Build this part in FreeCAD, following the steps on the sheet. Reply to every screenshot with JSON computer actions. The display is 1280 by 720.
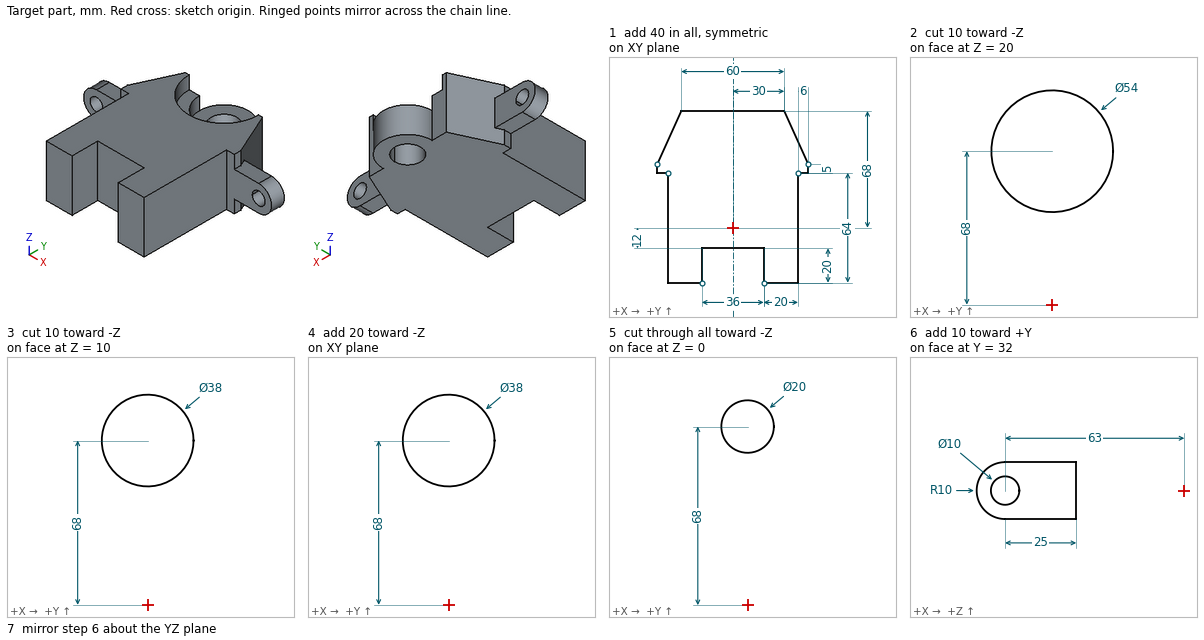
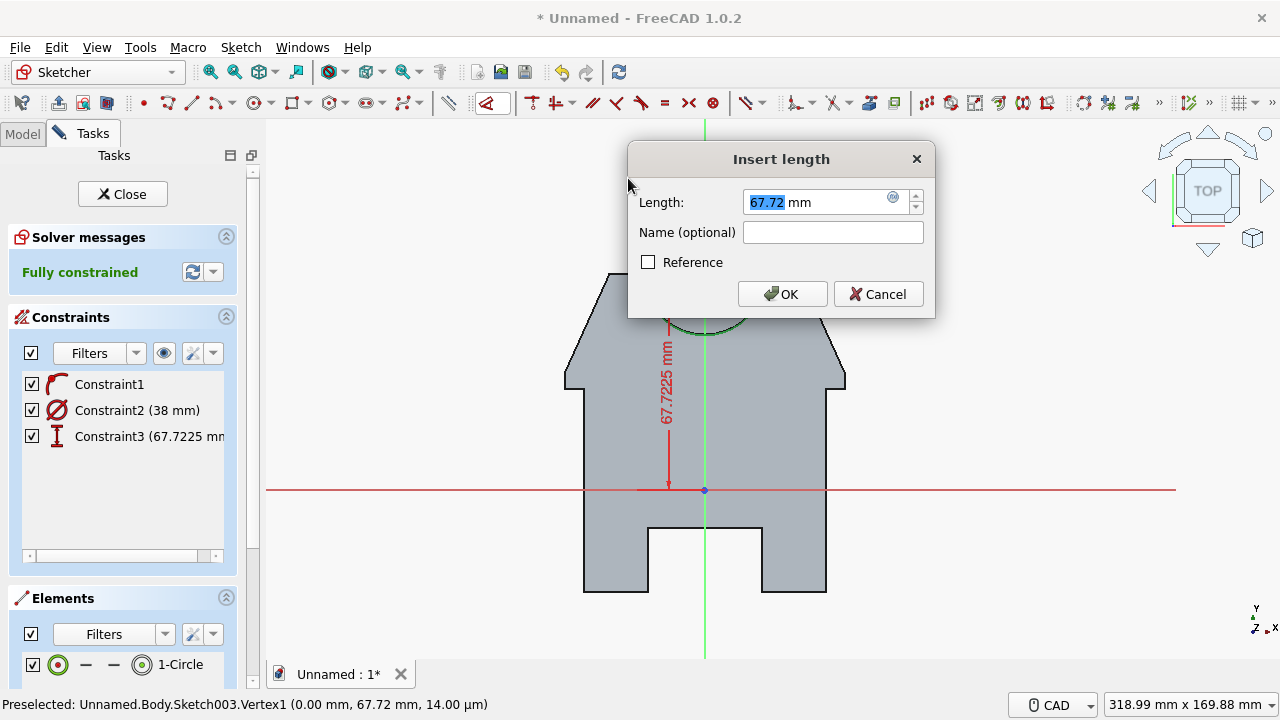
{"action": "type", "text": "68"}
{"action": "key", "text": "Return"}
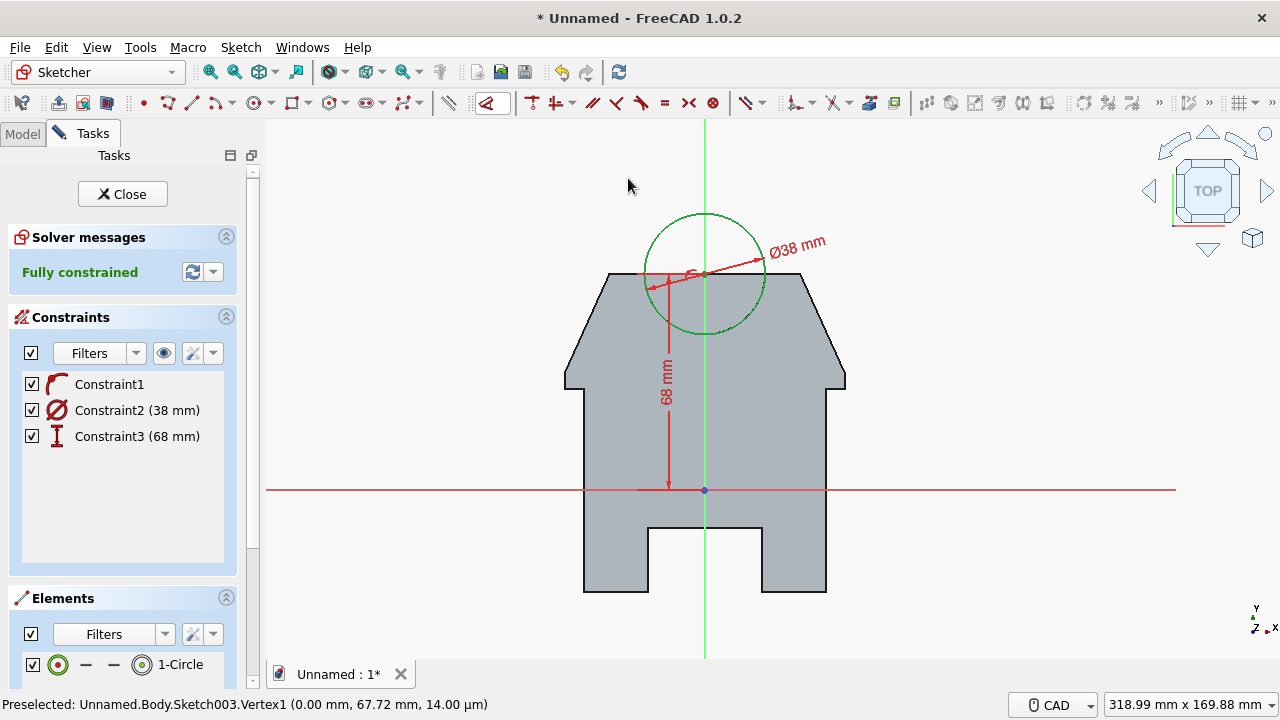
{"action": "left_click", "coordinate": [123, 194]}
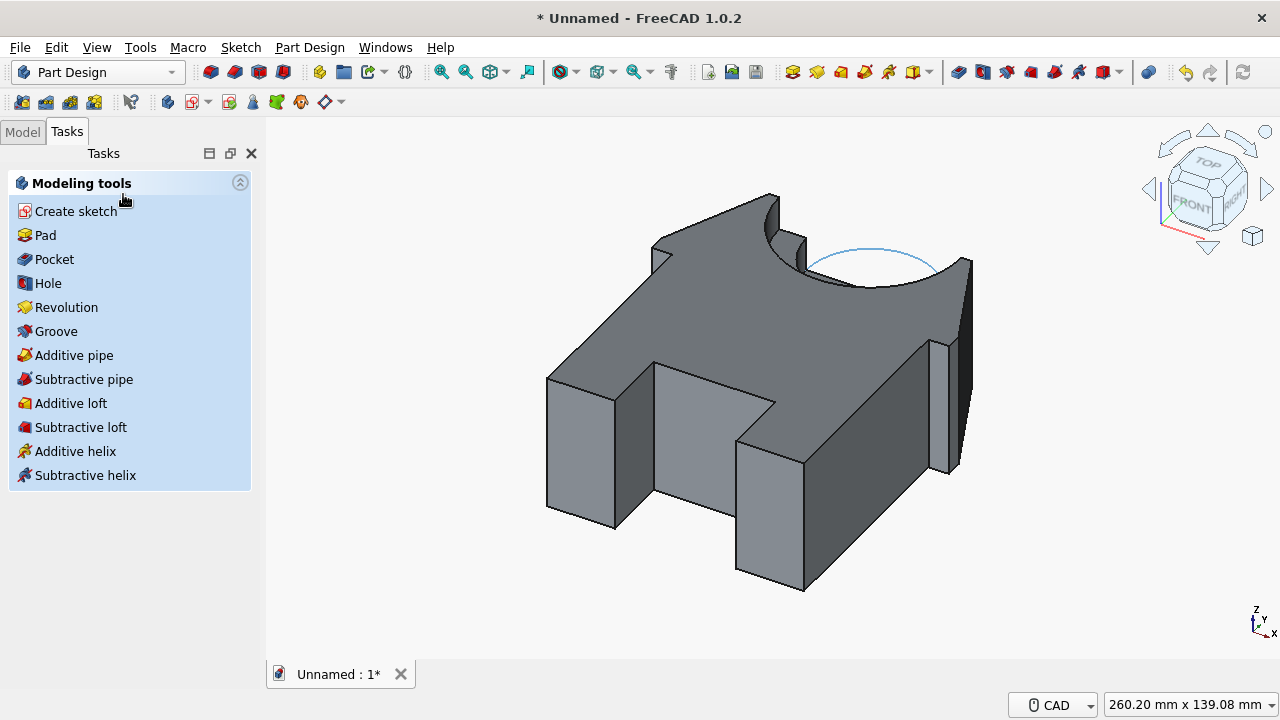
{"action": "left_click", "coordinate": [794, 72]}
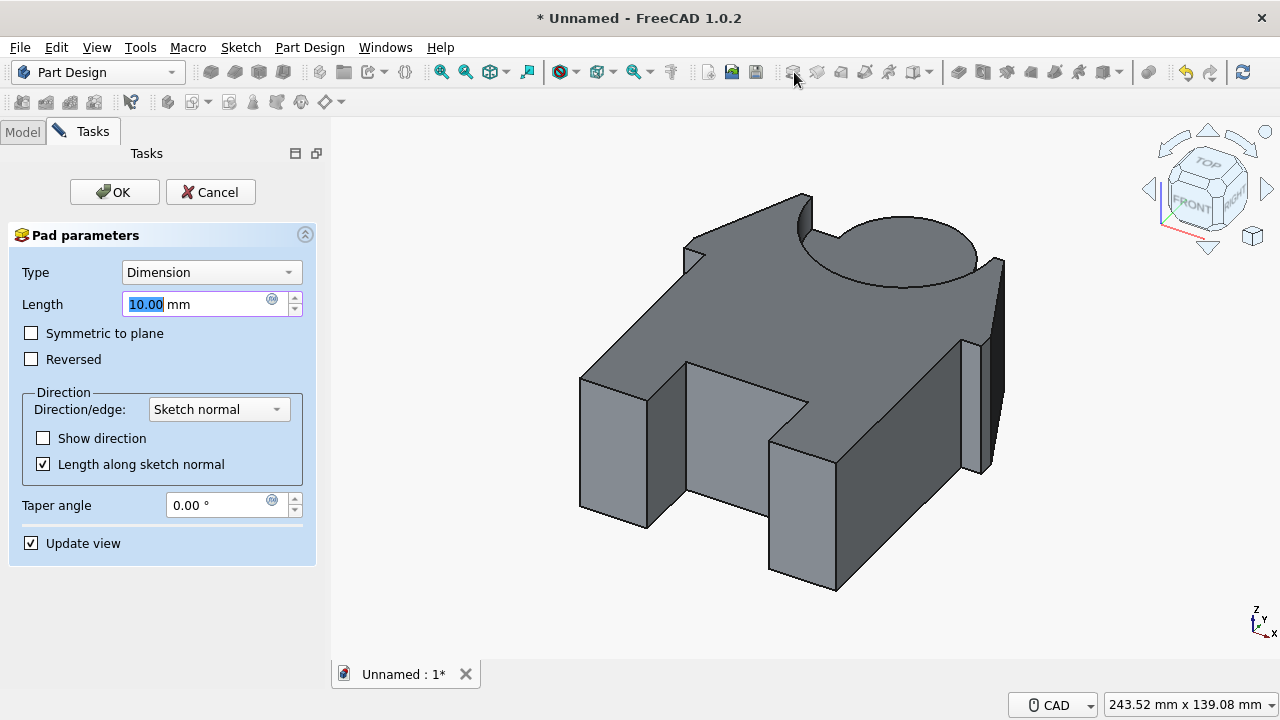
{"action": "type", "text": "20"}
{"action": "key", "text": "Tab"}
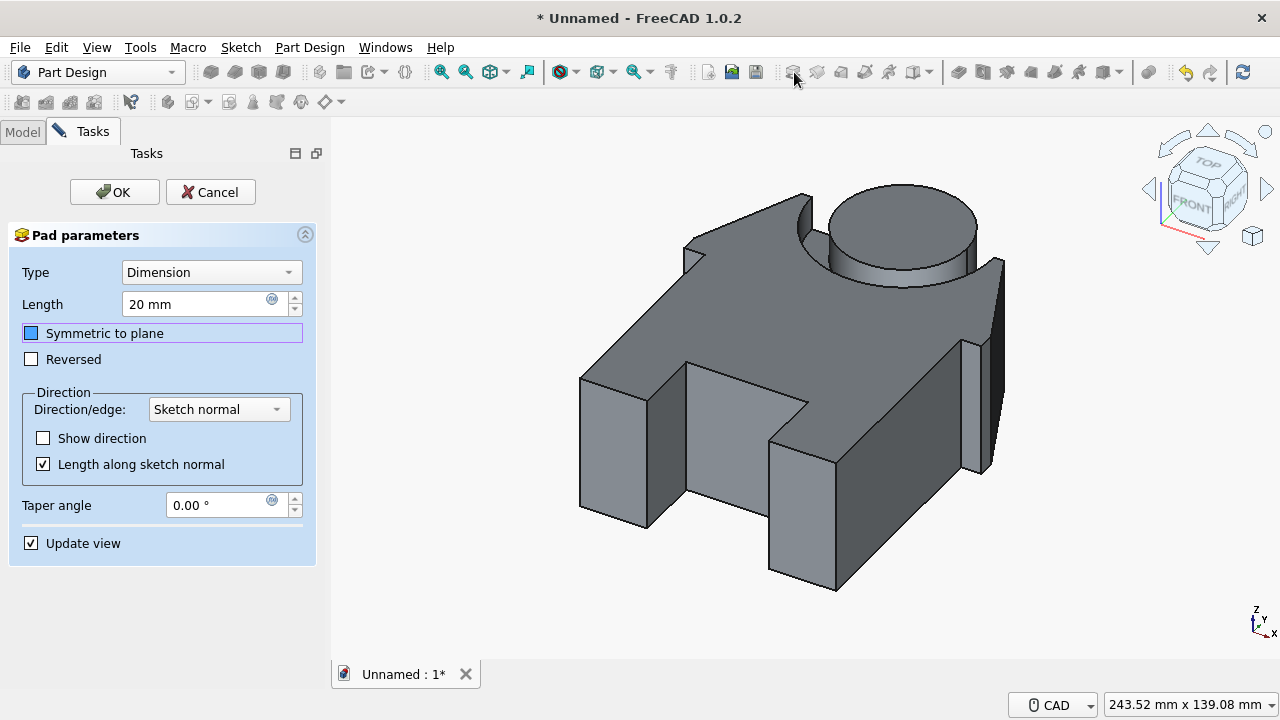
{"action": "left_click", "coordinate": [30, 359]}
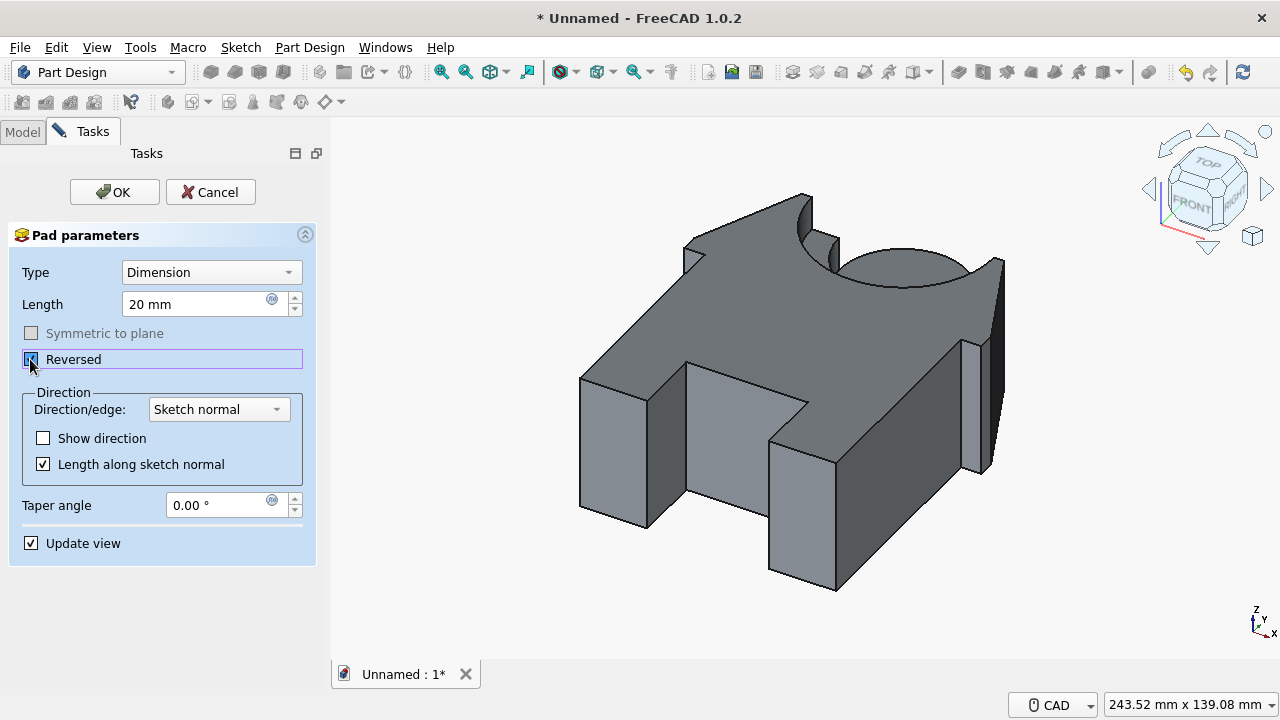
{"action": "left_click", "coordinate": [115, 192]}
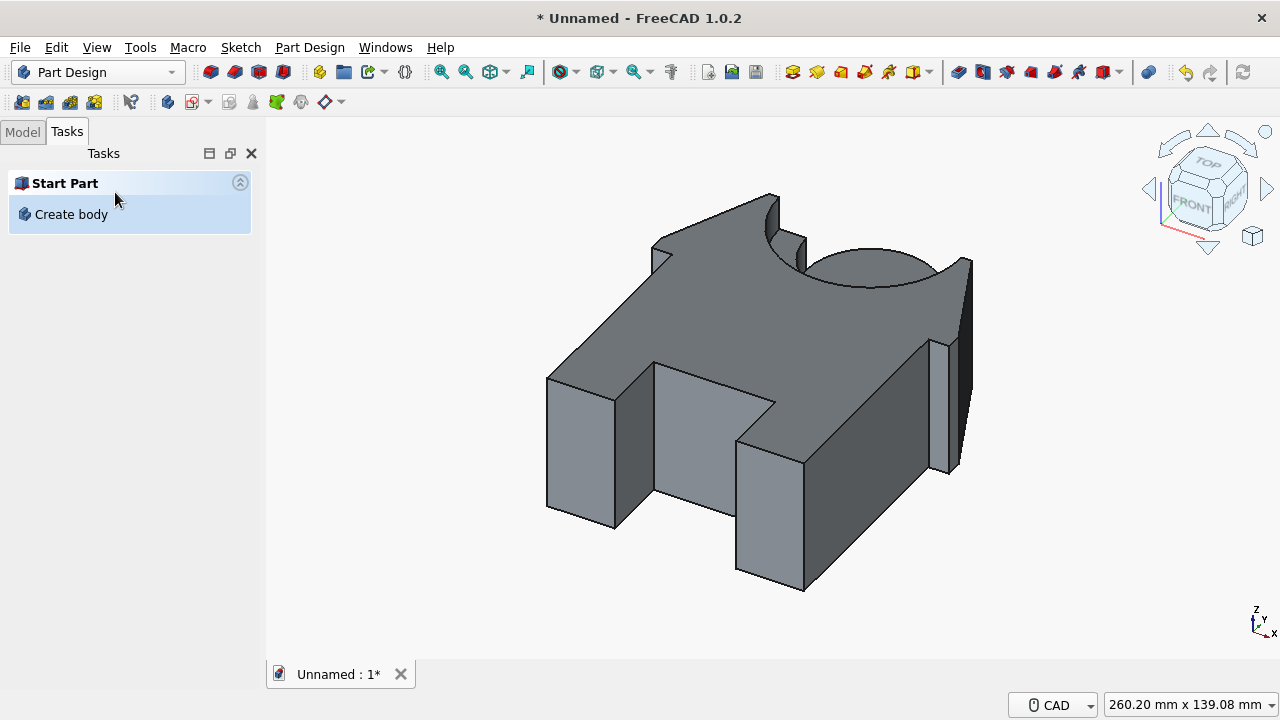
{"action": "key", "text": "0"}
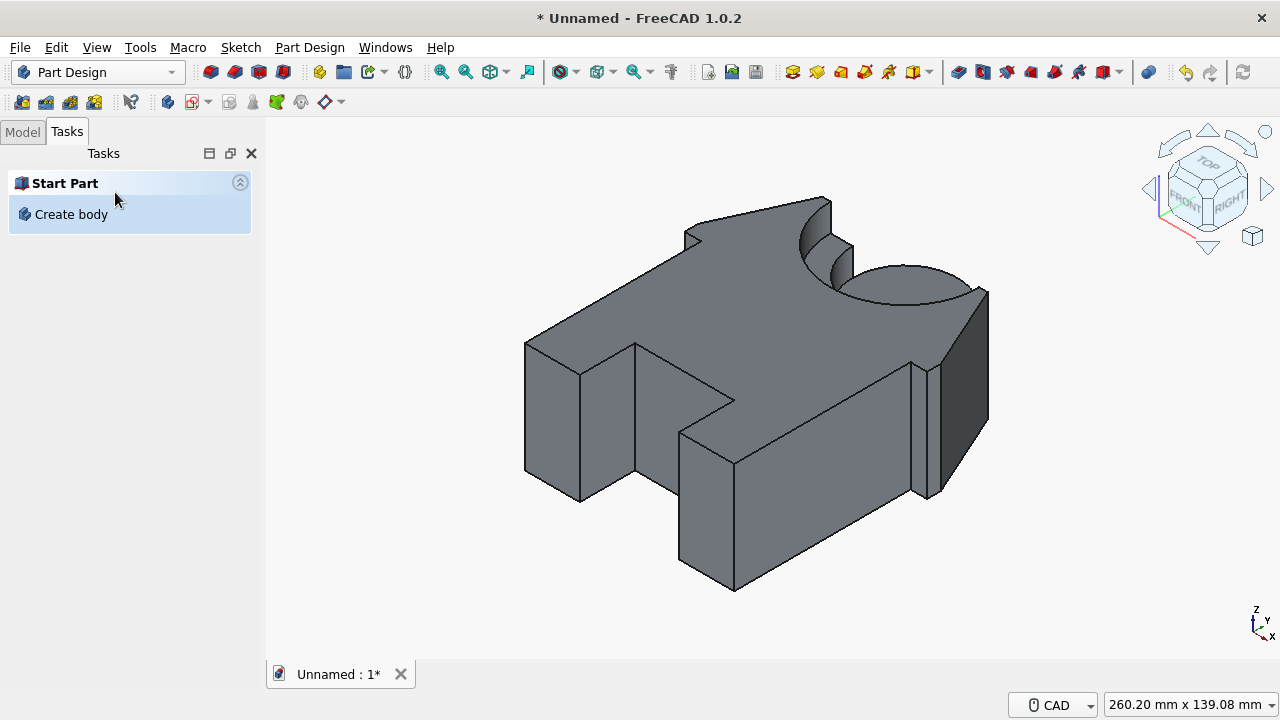
{"action": "key", "text": "2"}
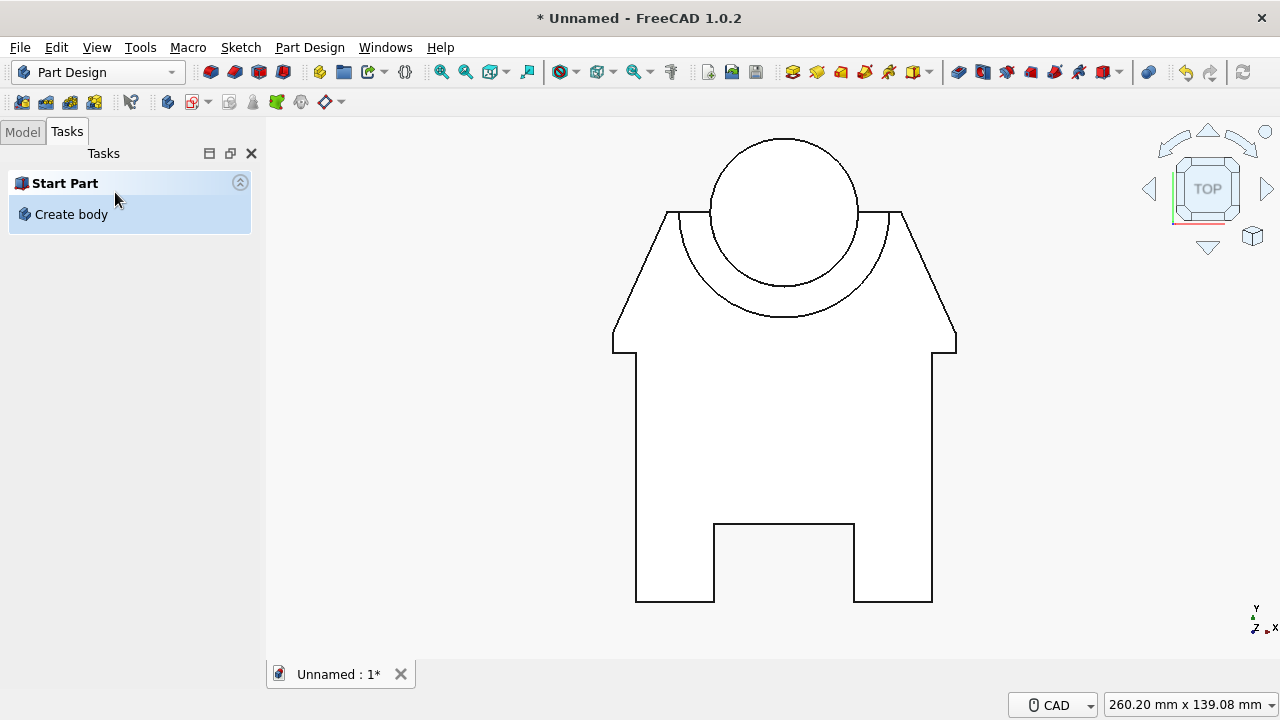
{"action": "left_click", "coordinate": [784, 211]}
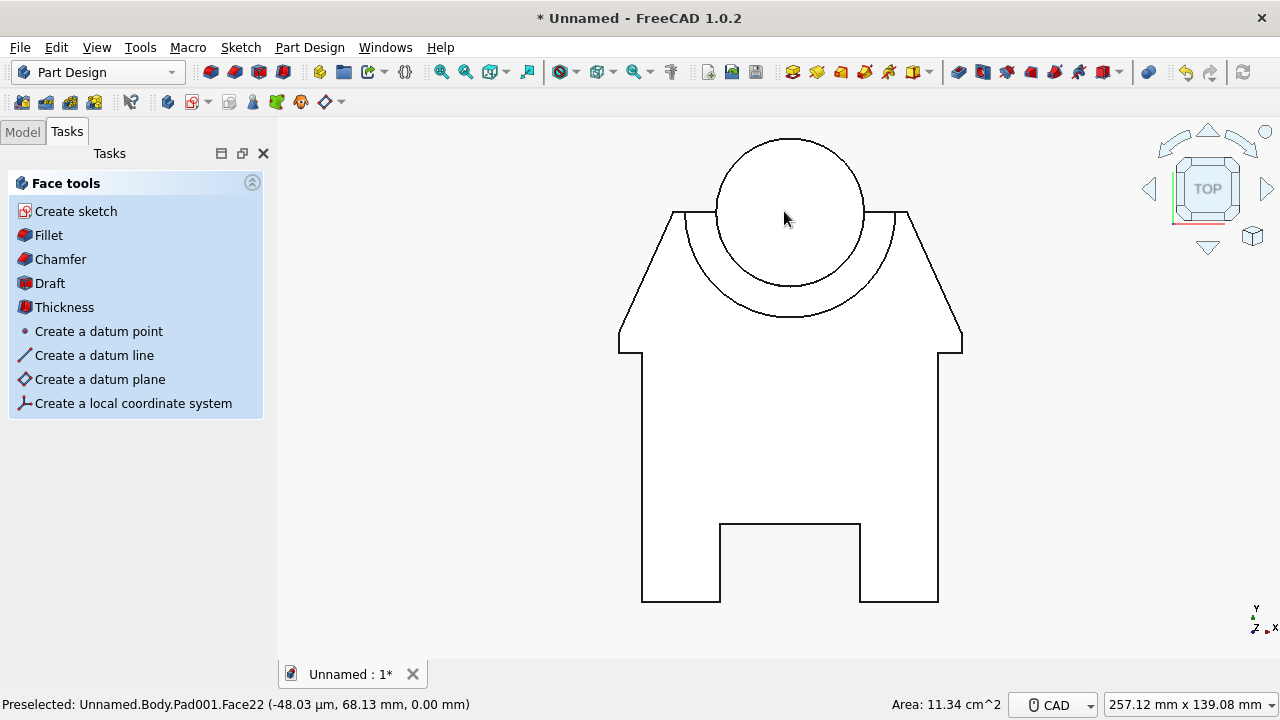
{"action": "left_click", "coordinate": [192, 102]}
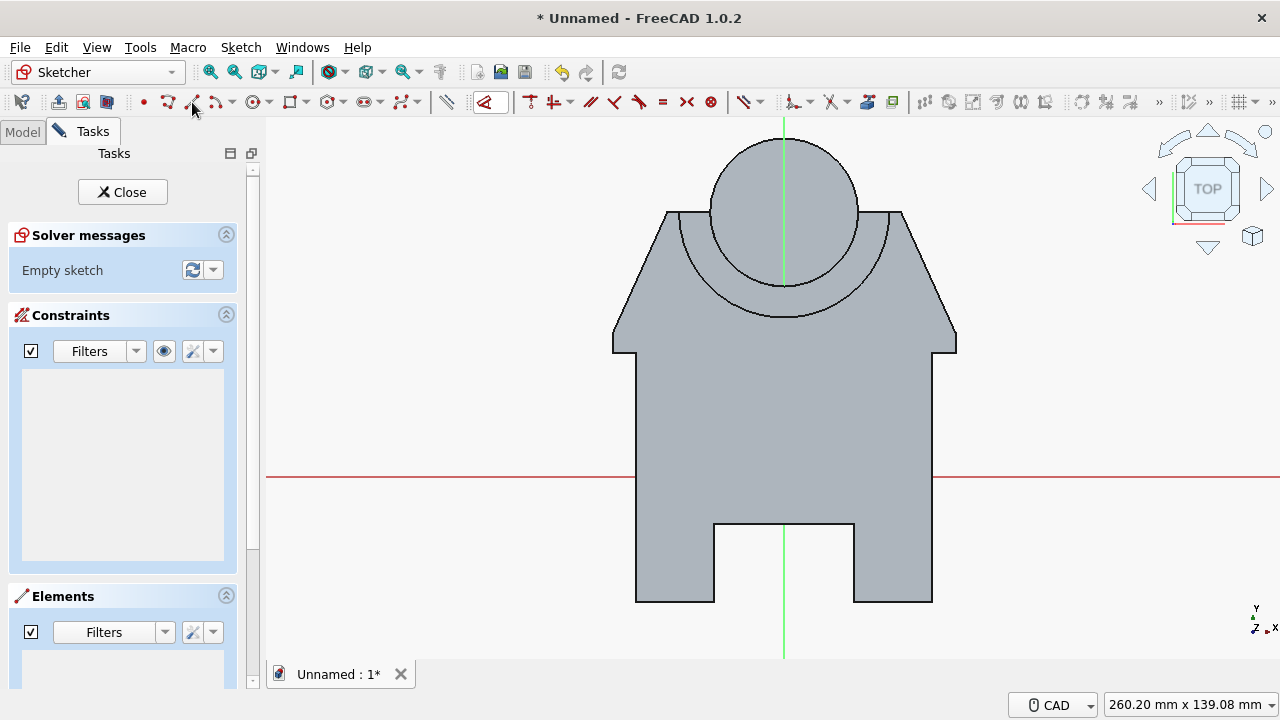
{"action": "scroll", "coordinate": [810, 155], "scroll_direction": "up", "scroll_amount": 7}